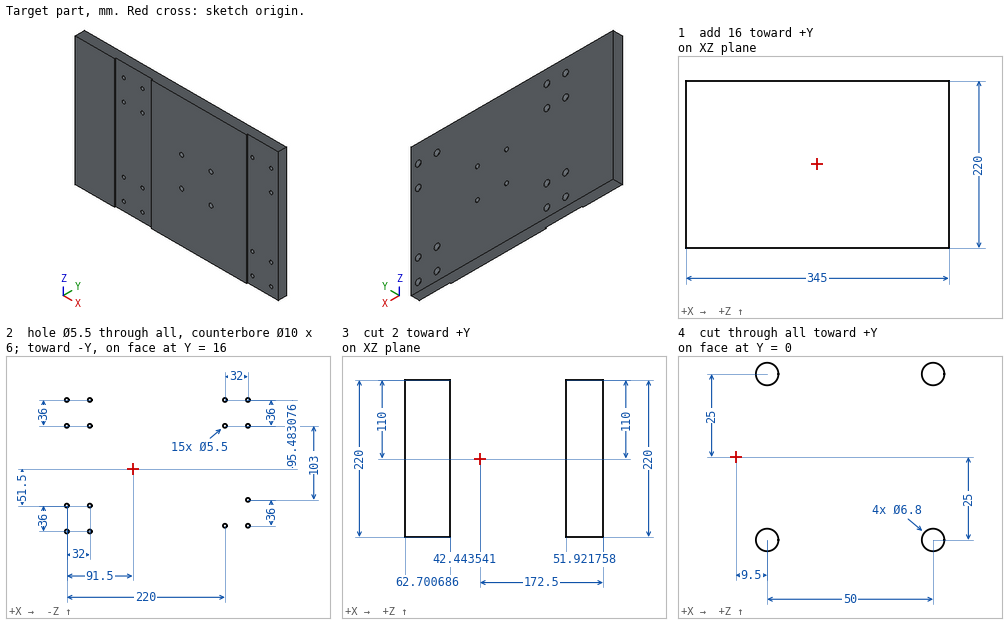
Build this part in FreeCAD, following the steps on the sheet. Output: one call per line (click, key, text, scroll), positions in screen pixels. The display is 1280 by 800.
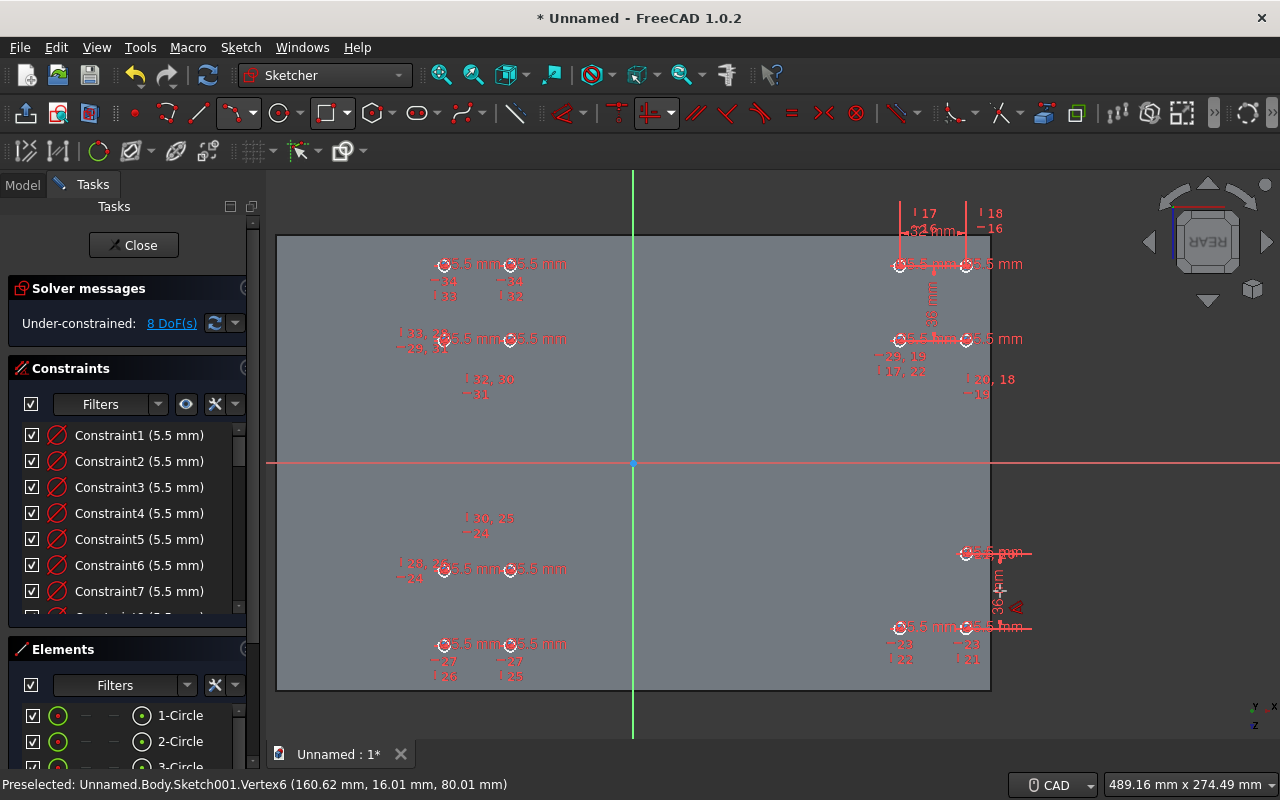
click(444, 571)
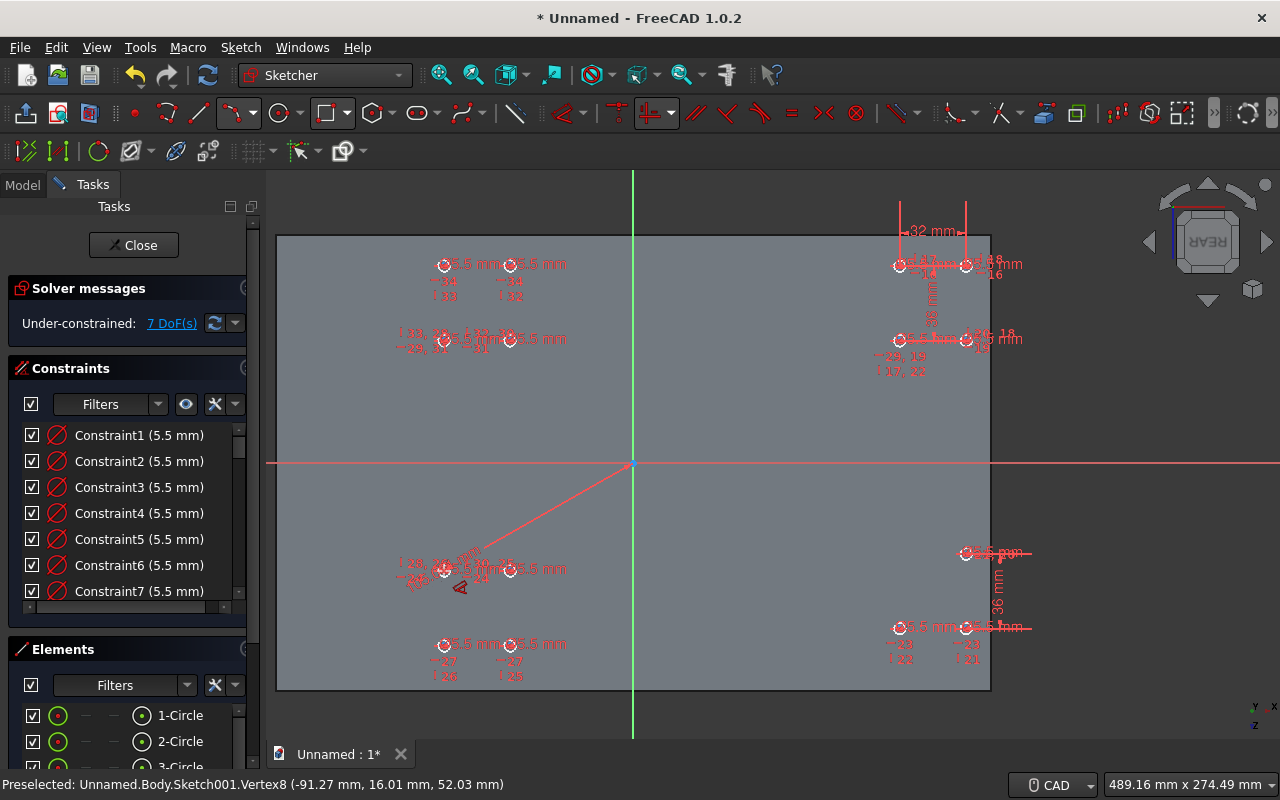
click(510, 571)
click(477, 605)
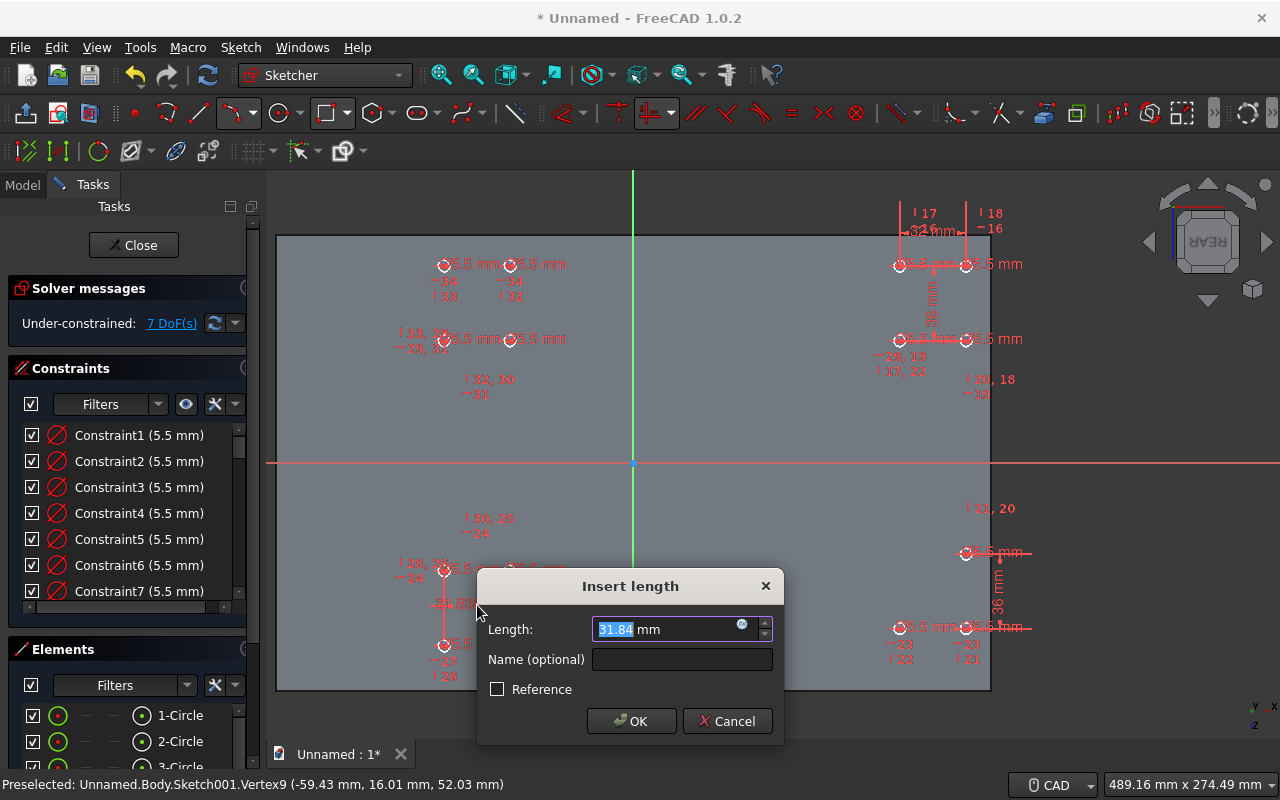
text(32)
key(Return)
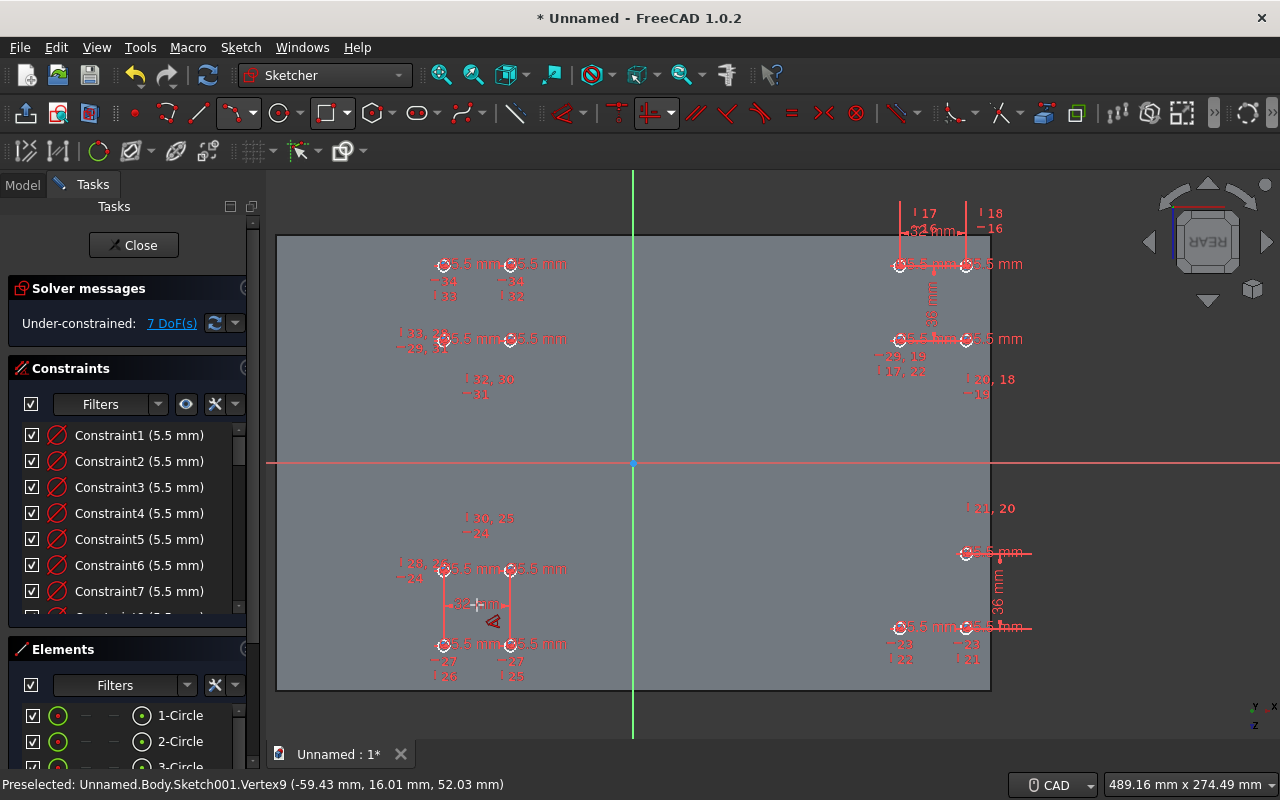
click(510, 571)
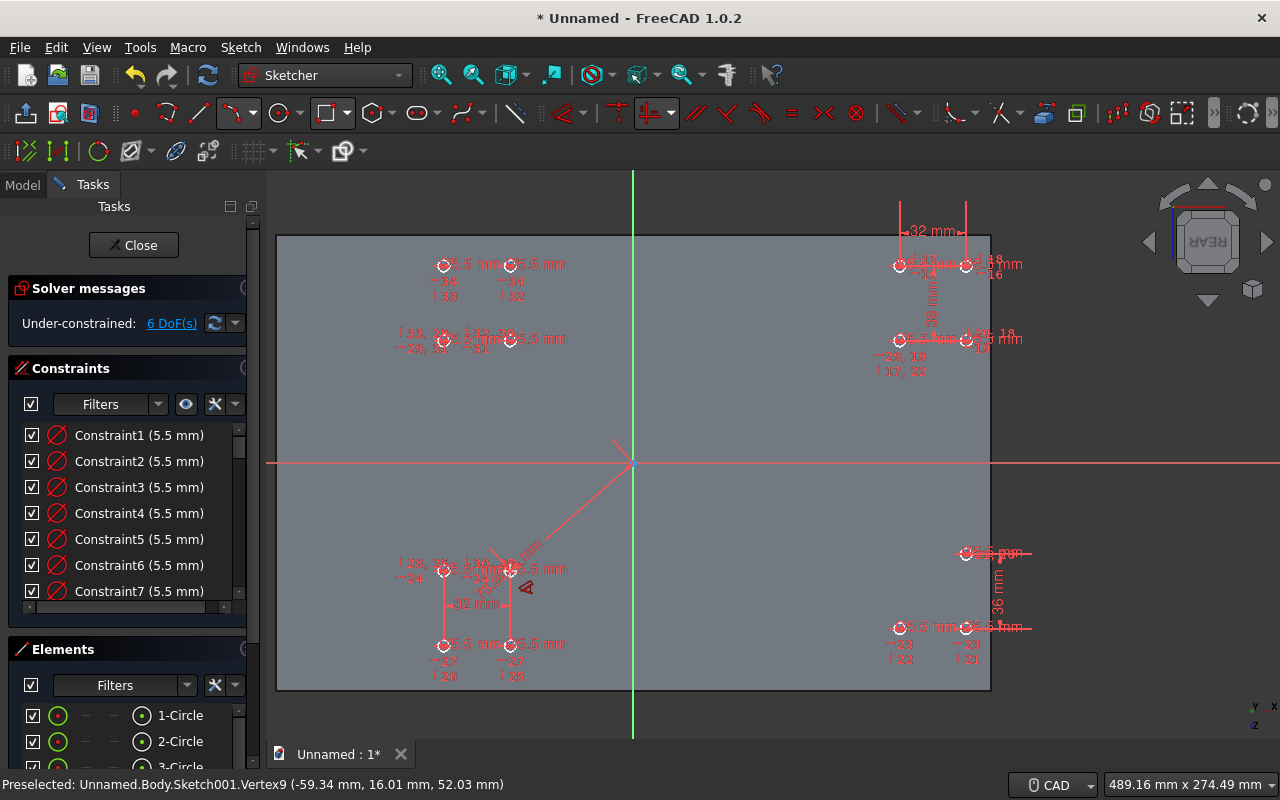
click(510, 646)
click(476, 626)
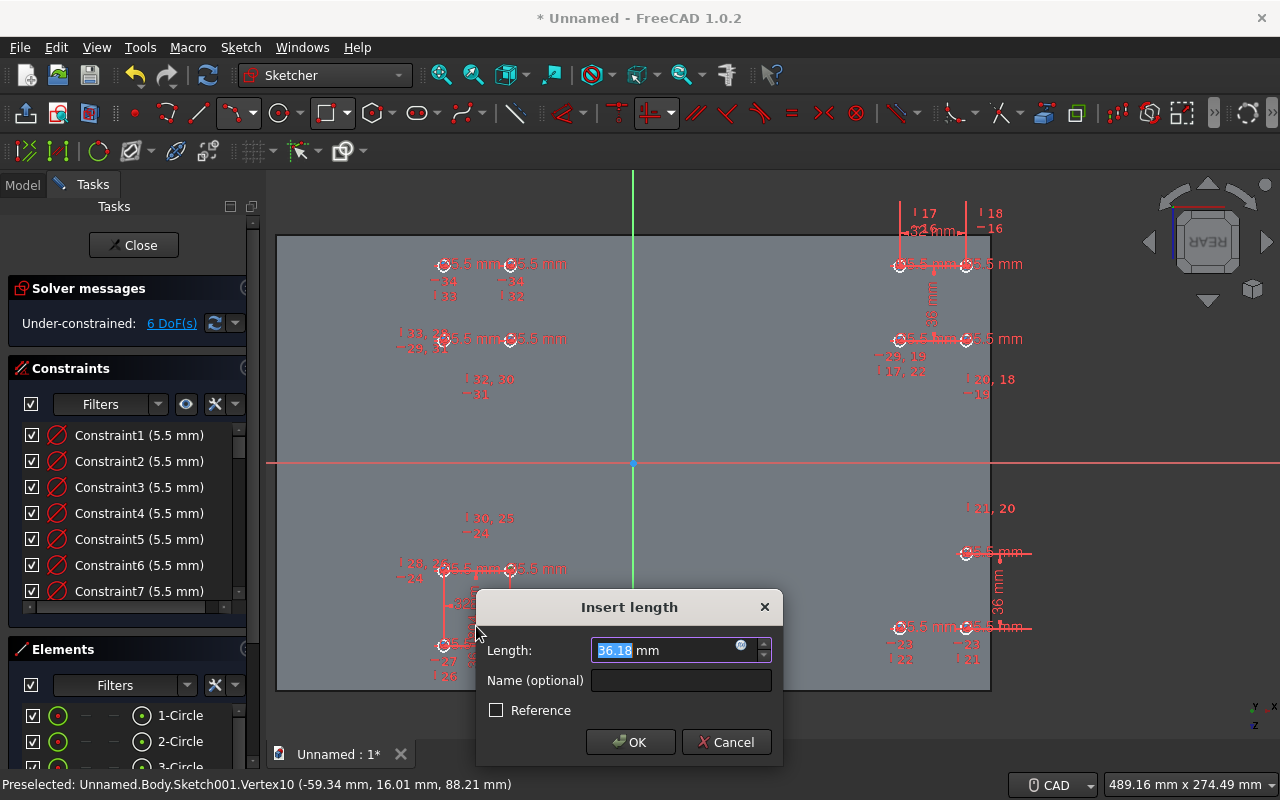
text(36)
key(Return)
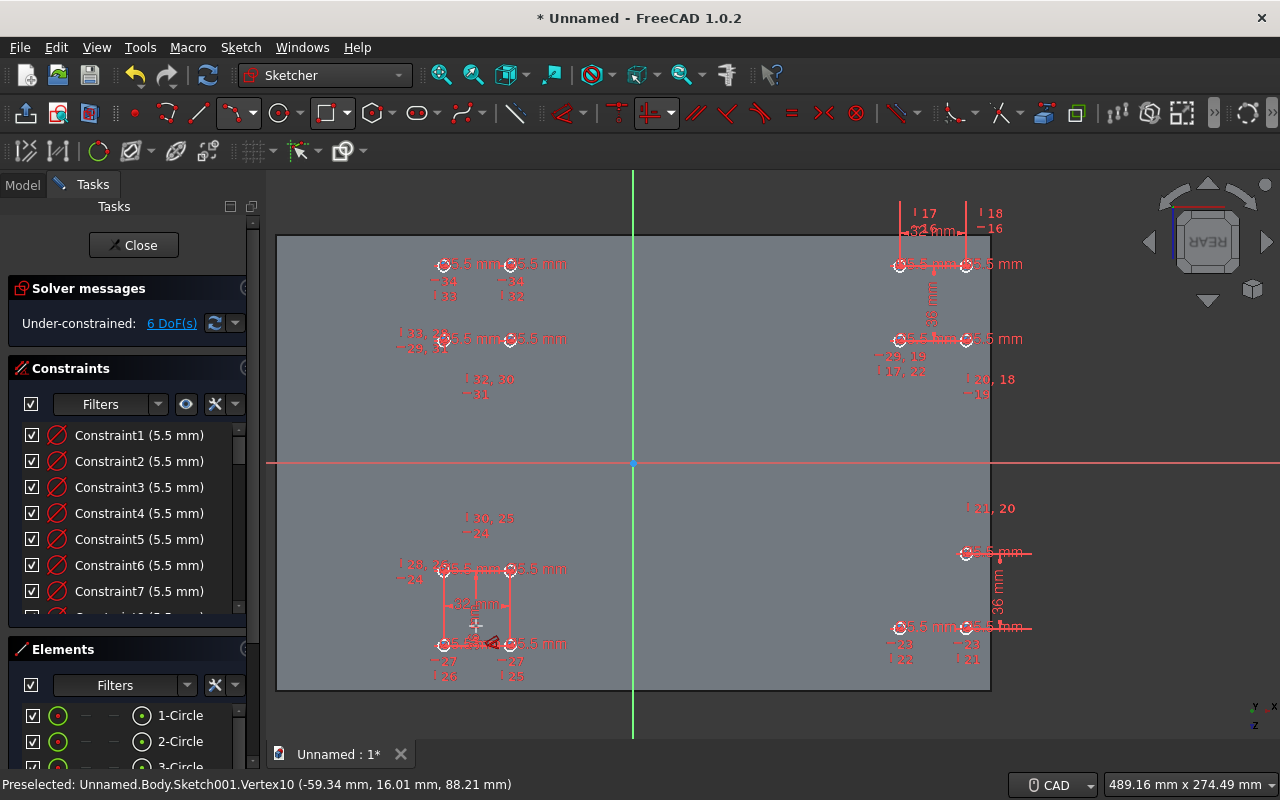
click(510, 341)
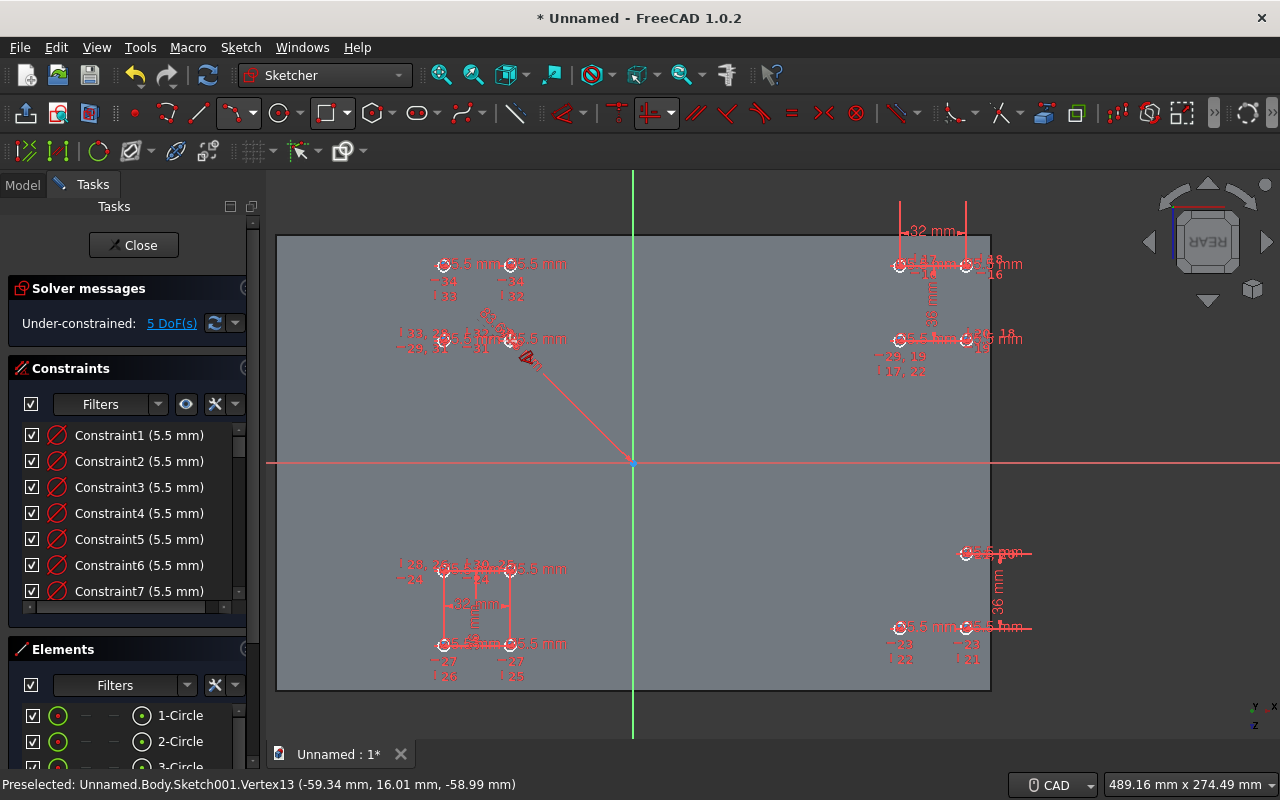
click(510, 266)
click(476, 303)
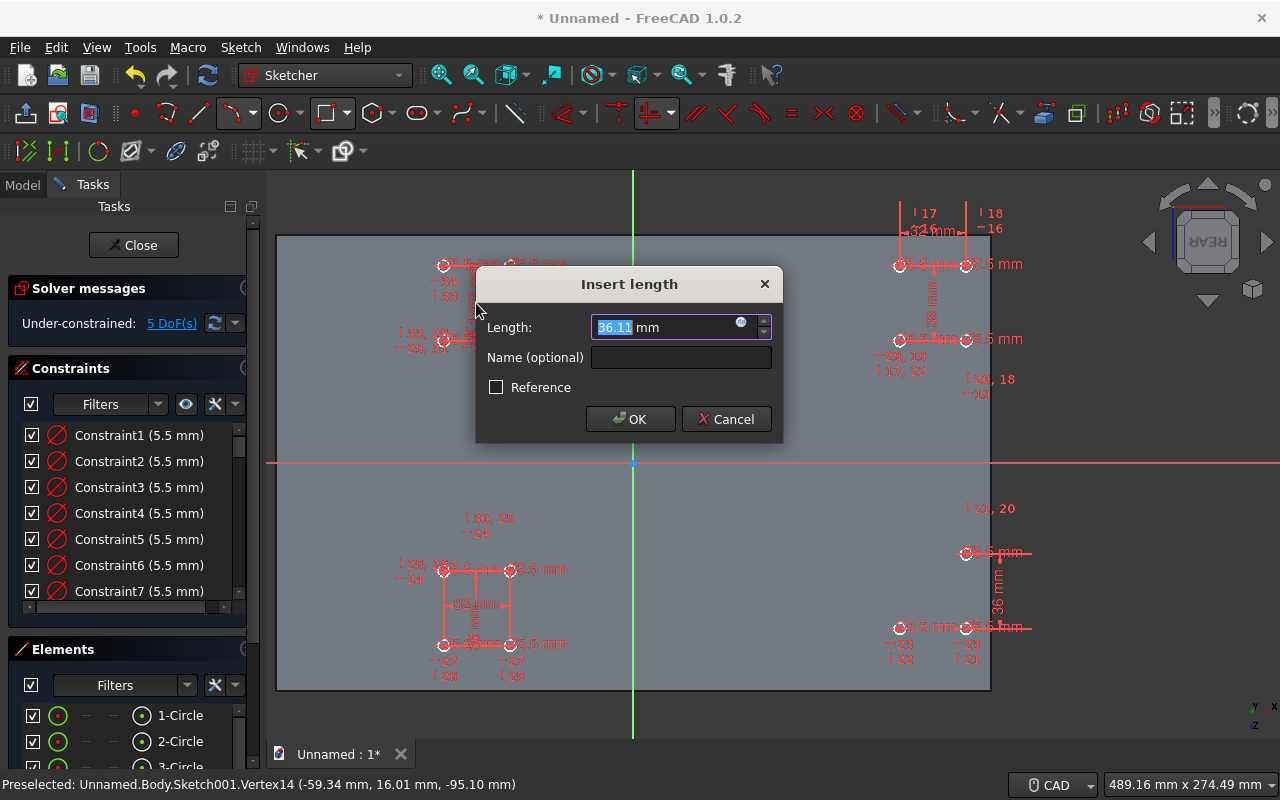
text(36)
key(Return)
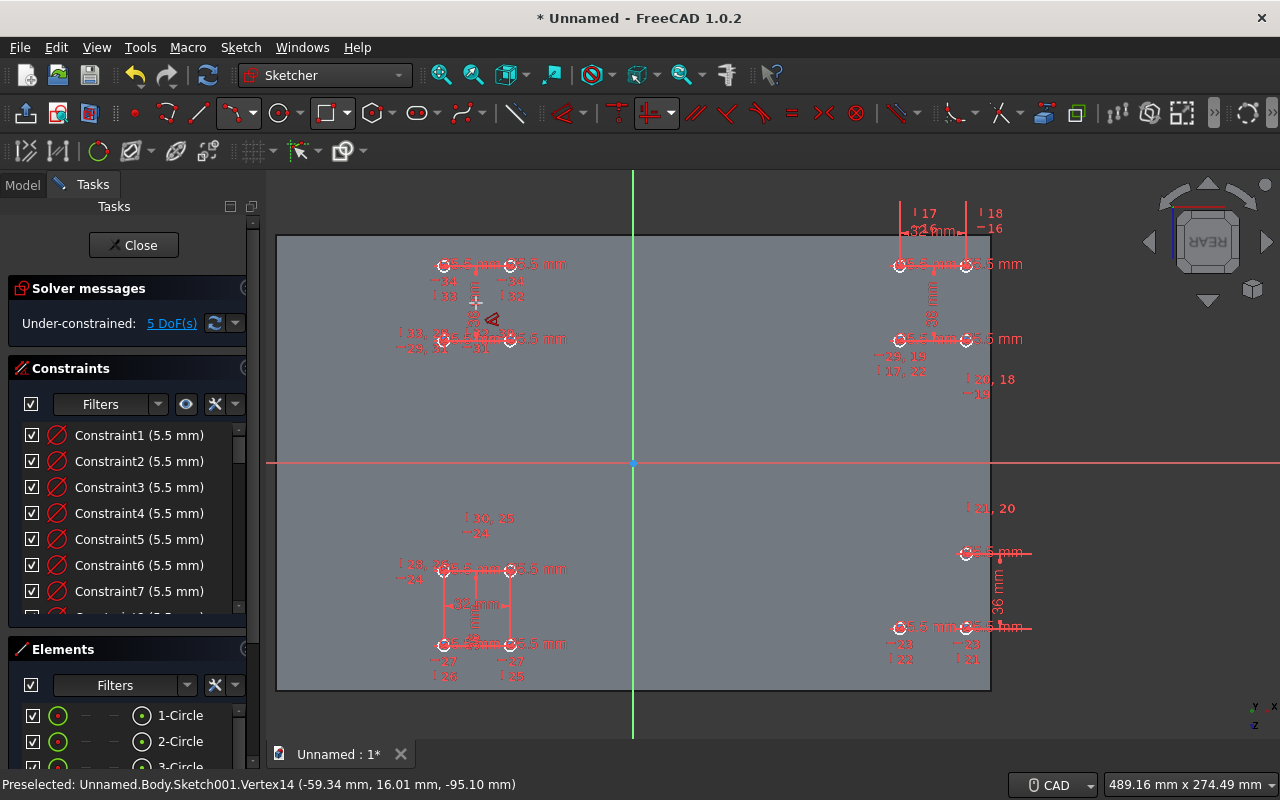
click(444, 571)
click(582, 605)